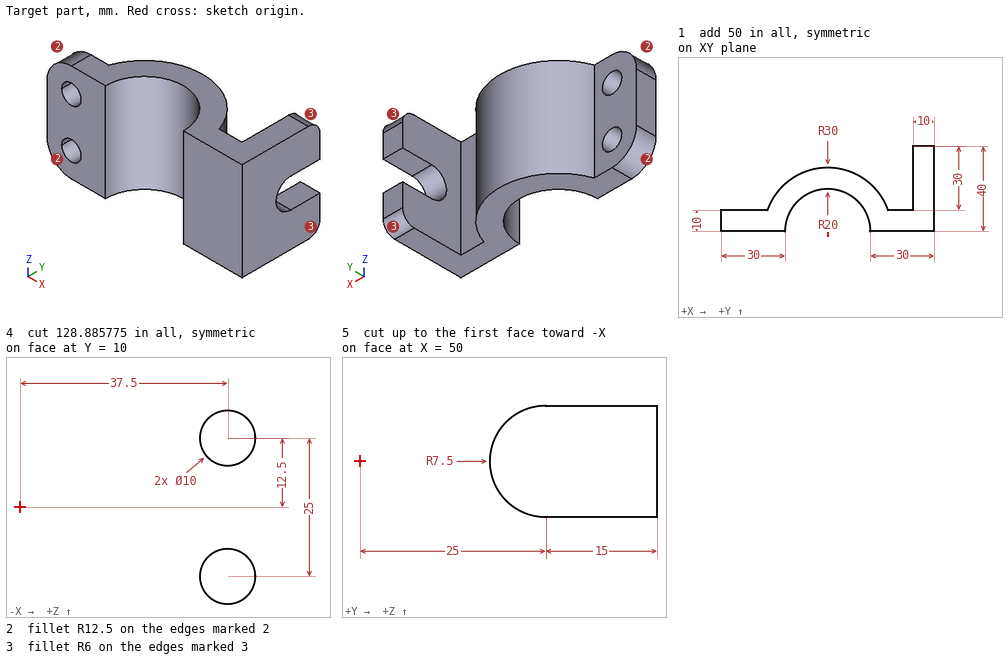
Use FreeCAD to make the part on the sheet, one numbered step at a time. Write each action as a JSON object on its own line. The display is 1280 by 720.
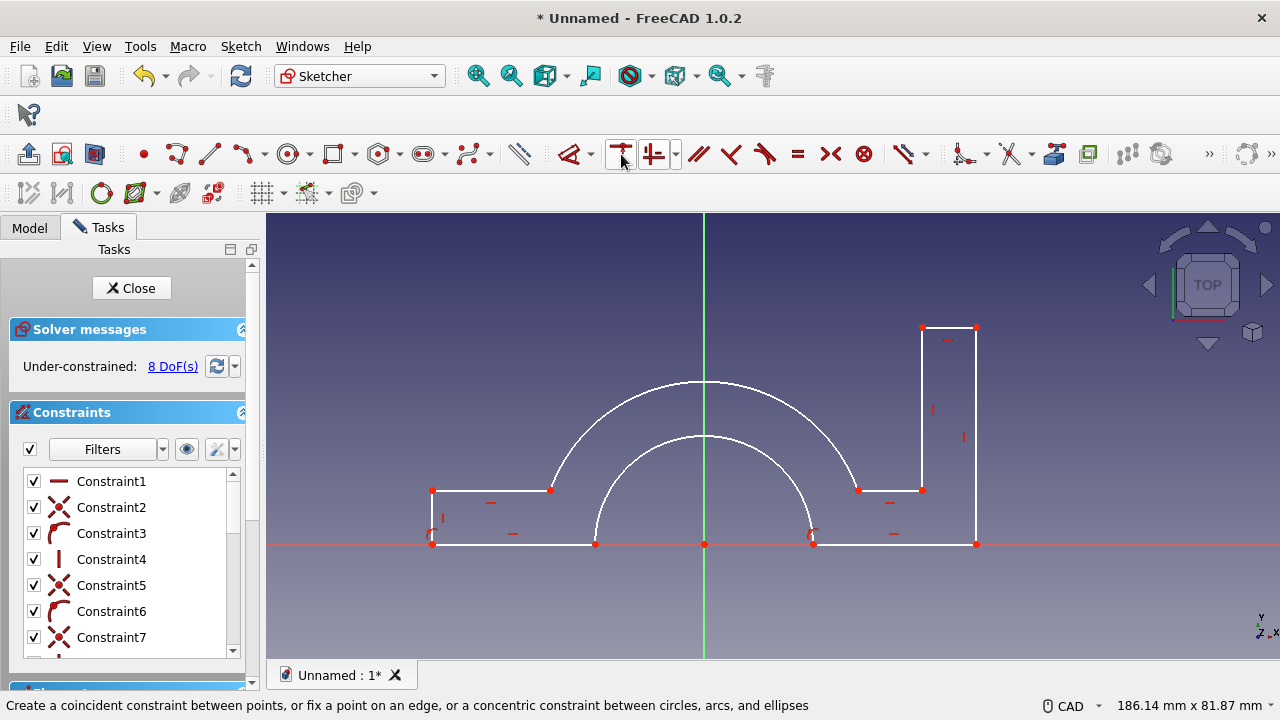
{"action": "left_click", "coordinate": [768, 457]}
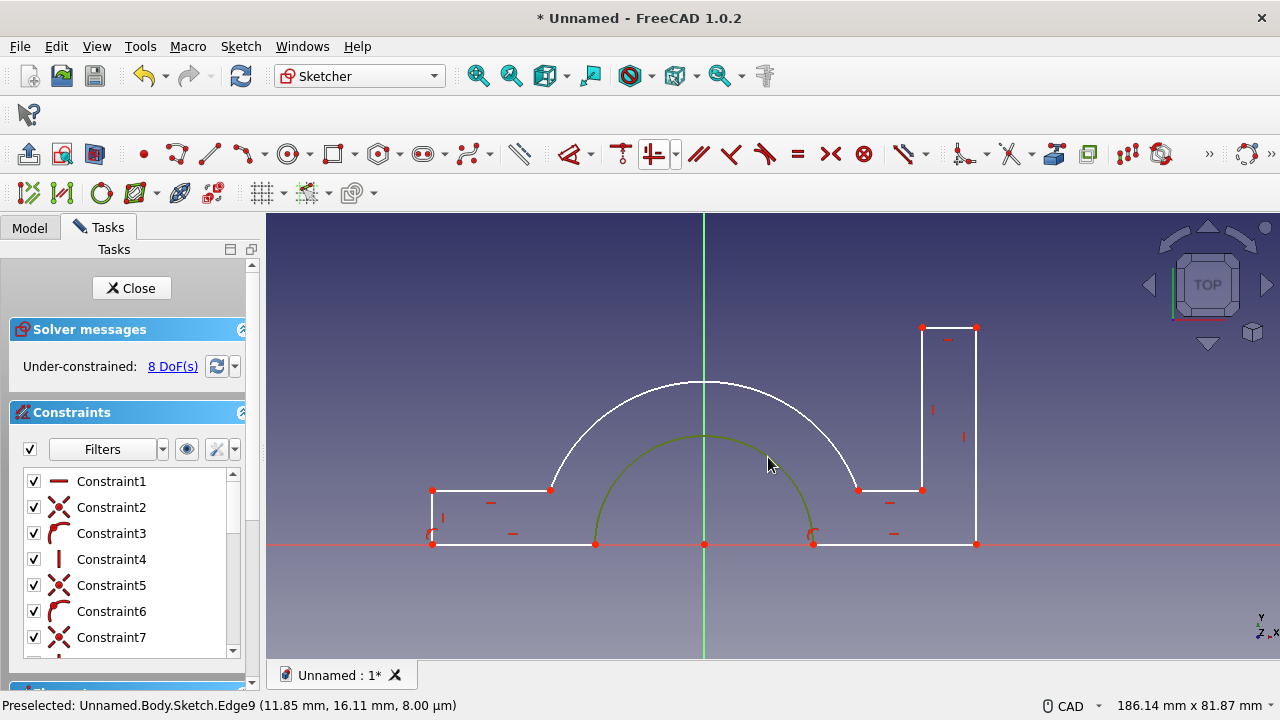
{"action": "key", "text": "k r"}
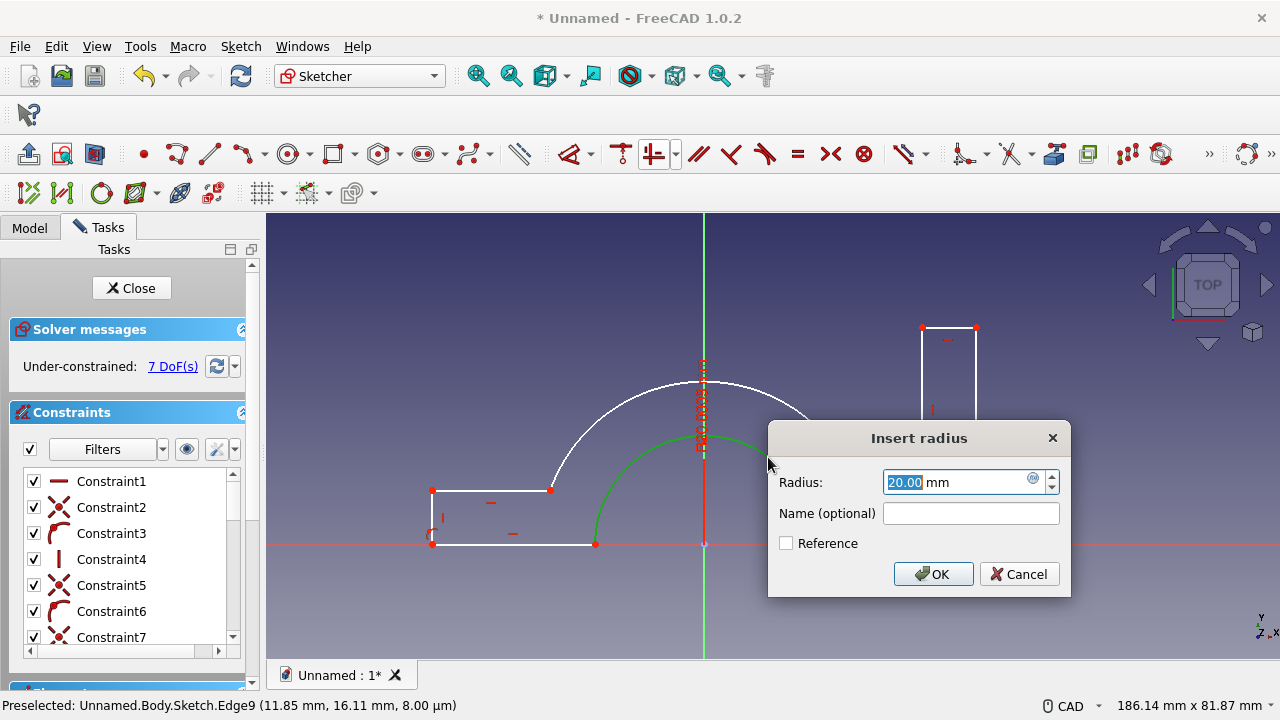
{"action": "type", "text": "20"}
{"action": "key", "text": "Return"}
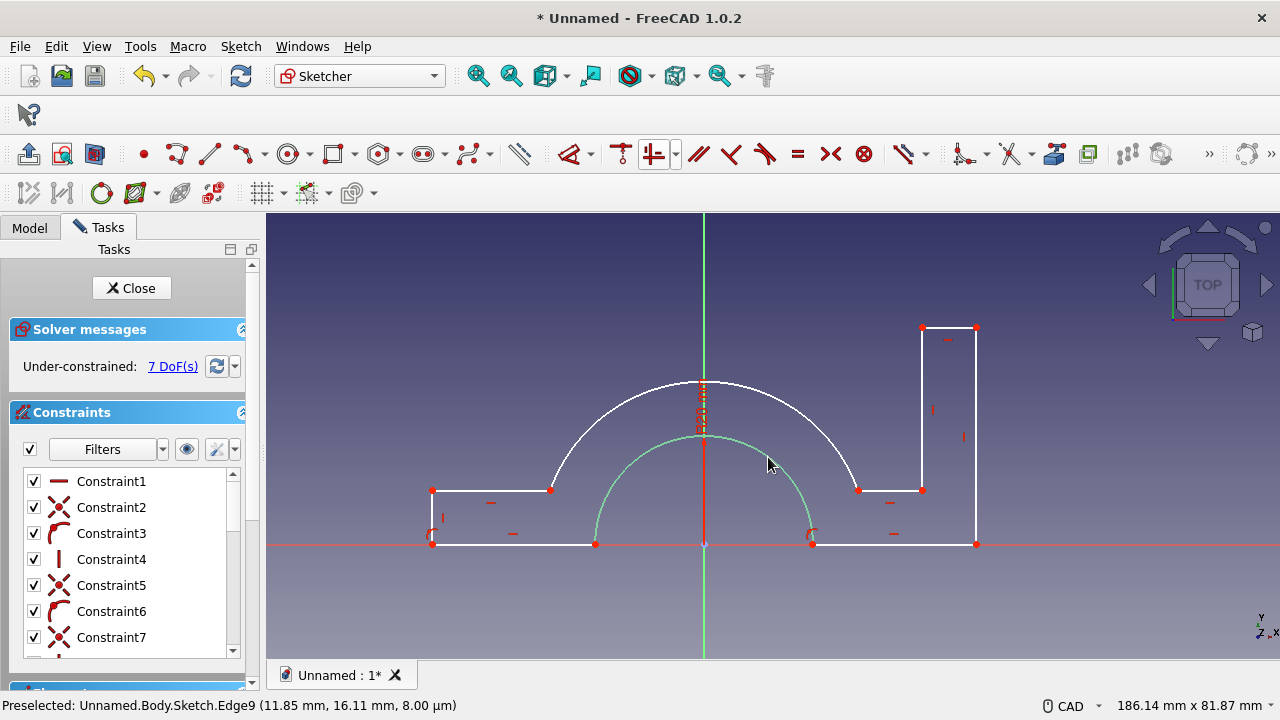
{"action": "left_click", "coordinate": [781, 401]}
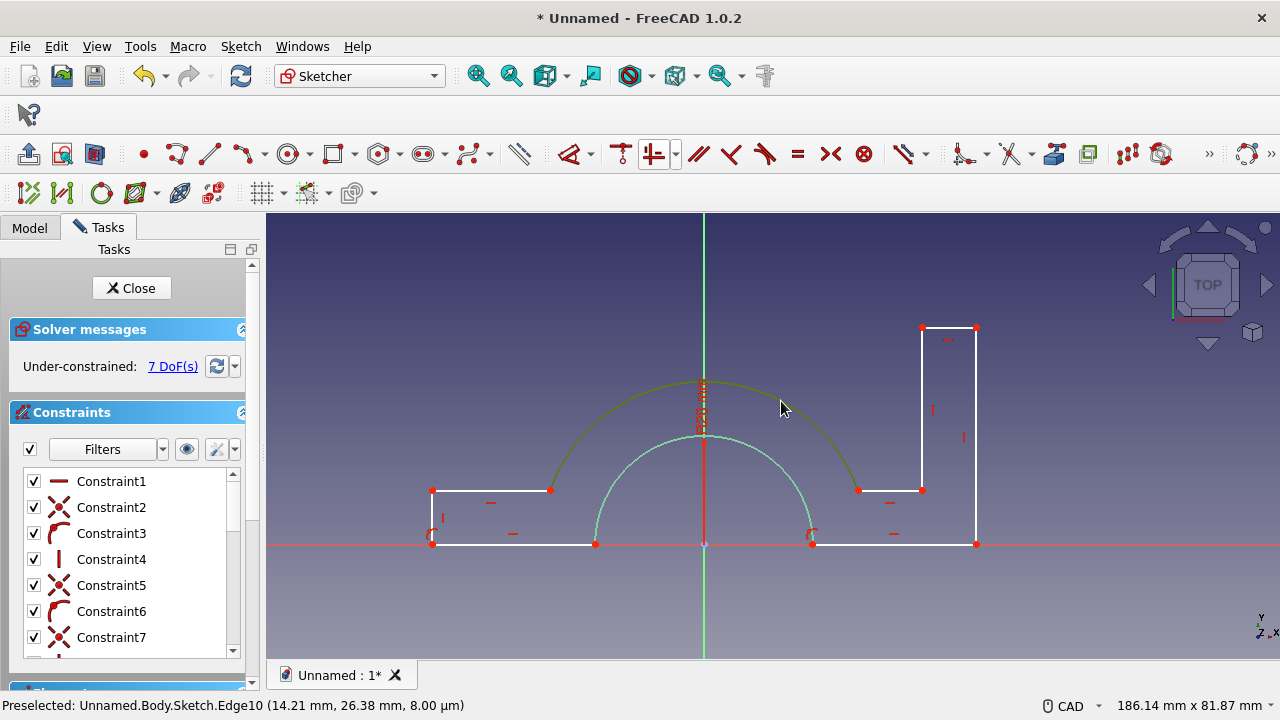
{"action": "left_click", "coordinate": [590, 154]}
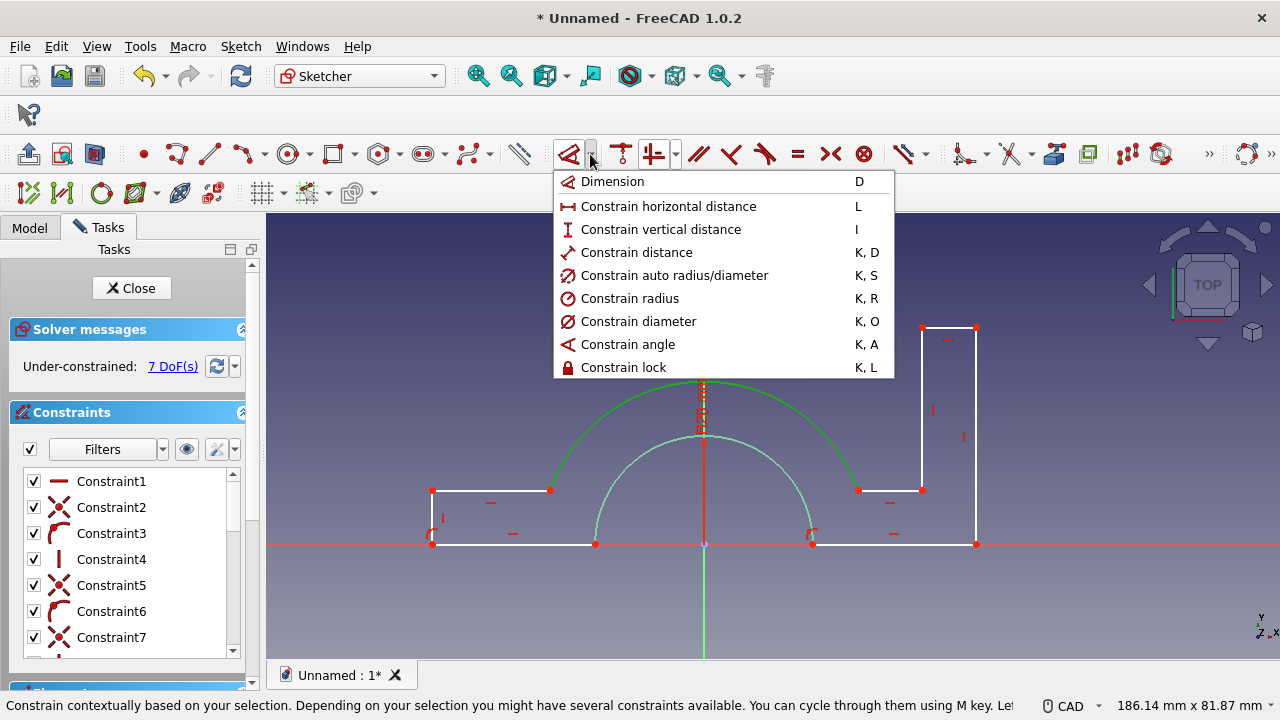
{"action": "left_click", "coordinate": [724, 298]}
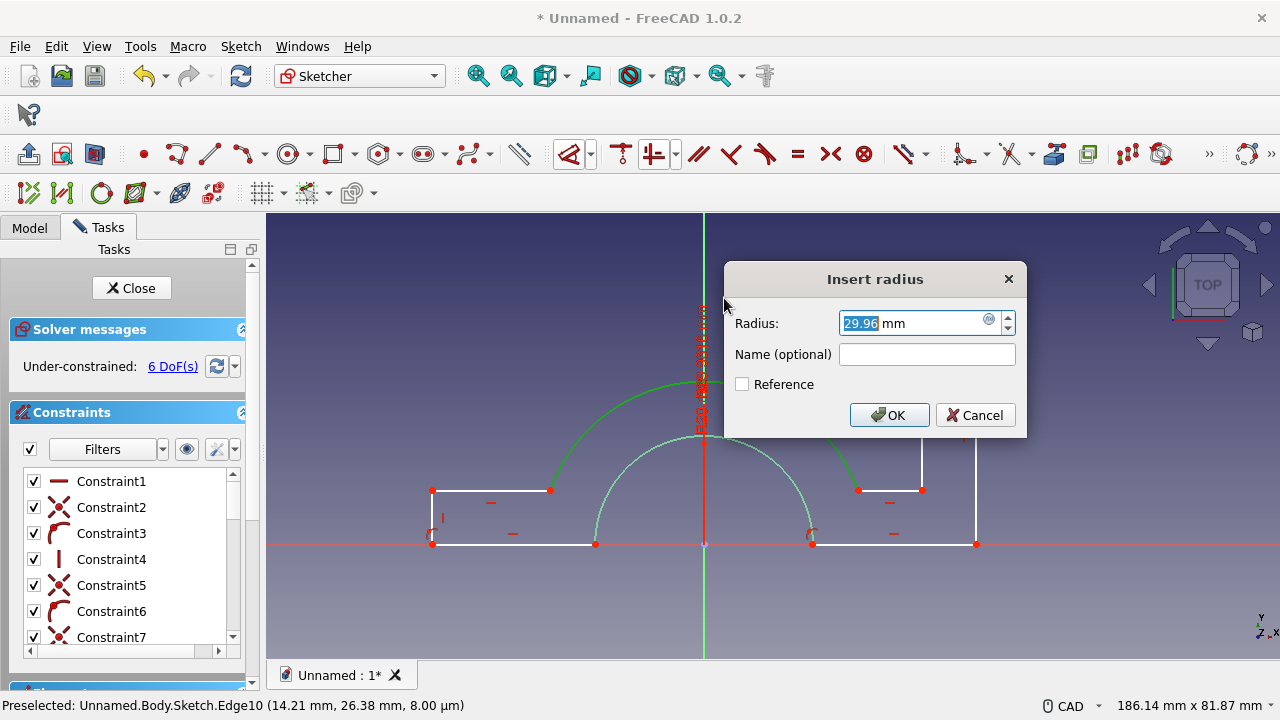
{"action": "type", "text": "30"}
{"action": "key", "text": "Return"}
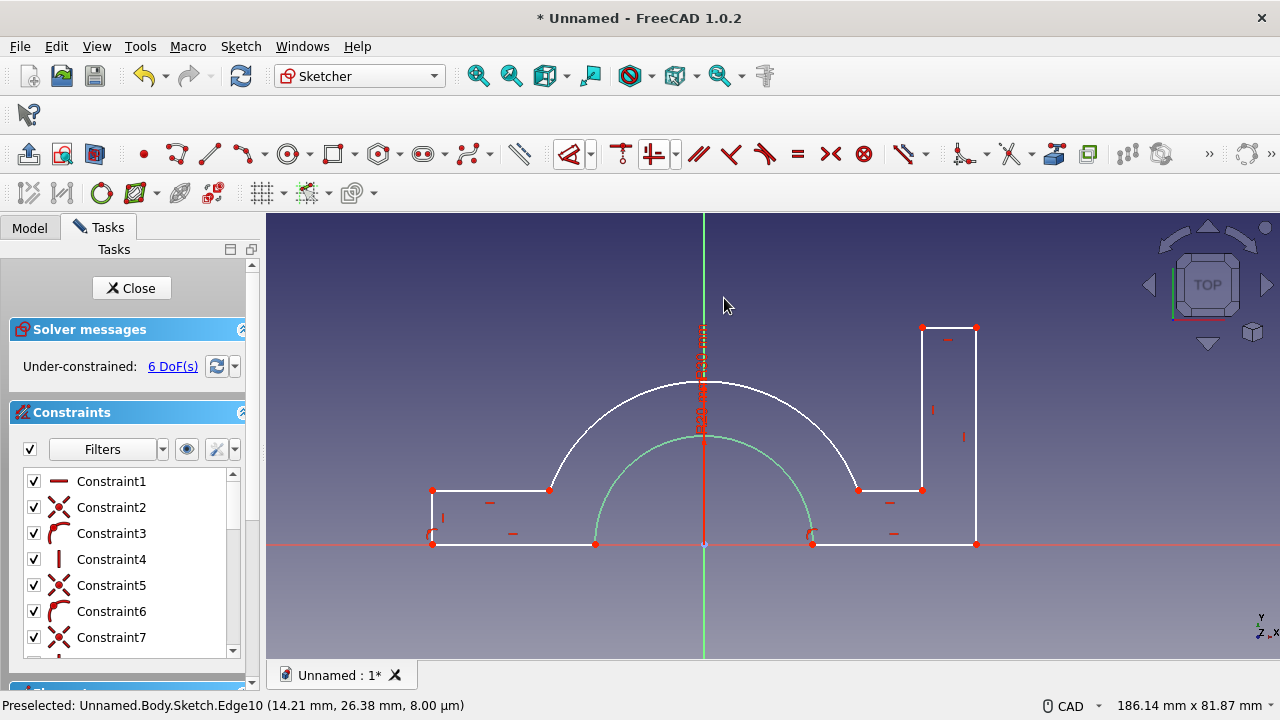
{"action": "left_click", "coordinate": [432, 507]}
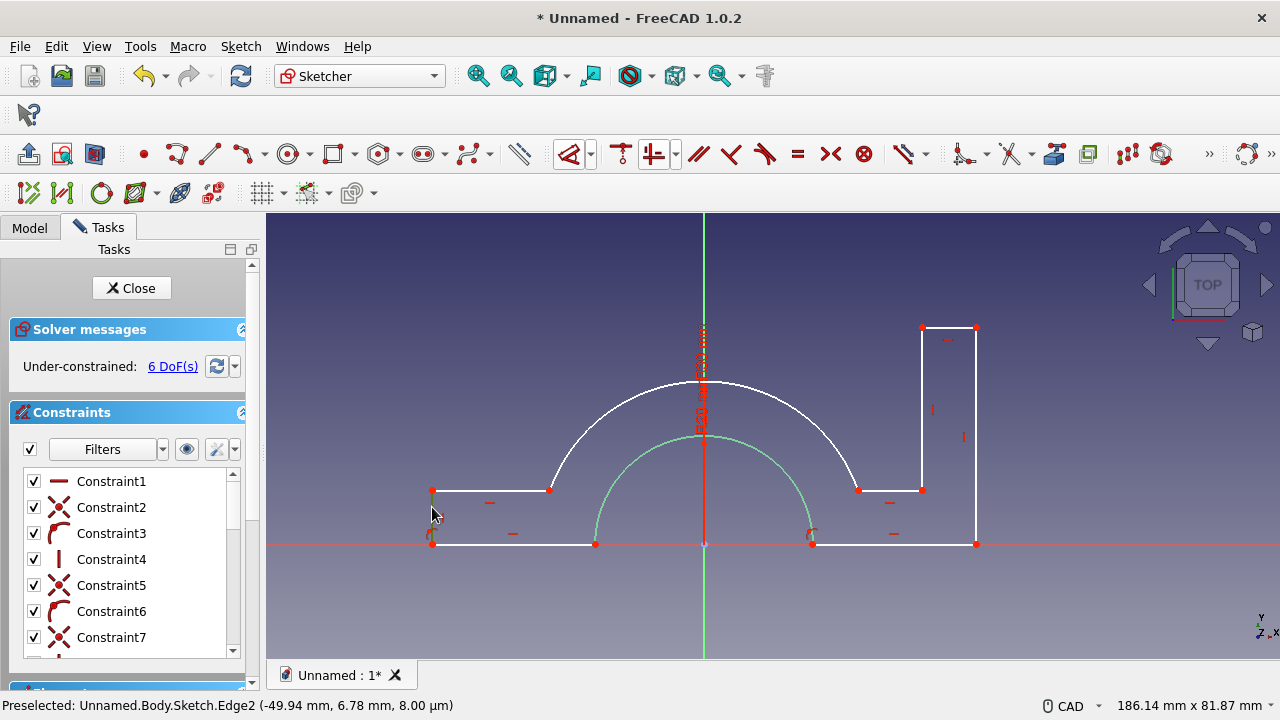
{"action": "key", "text": "i"}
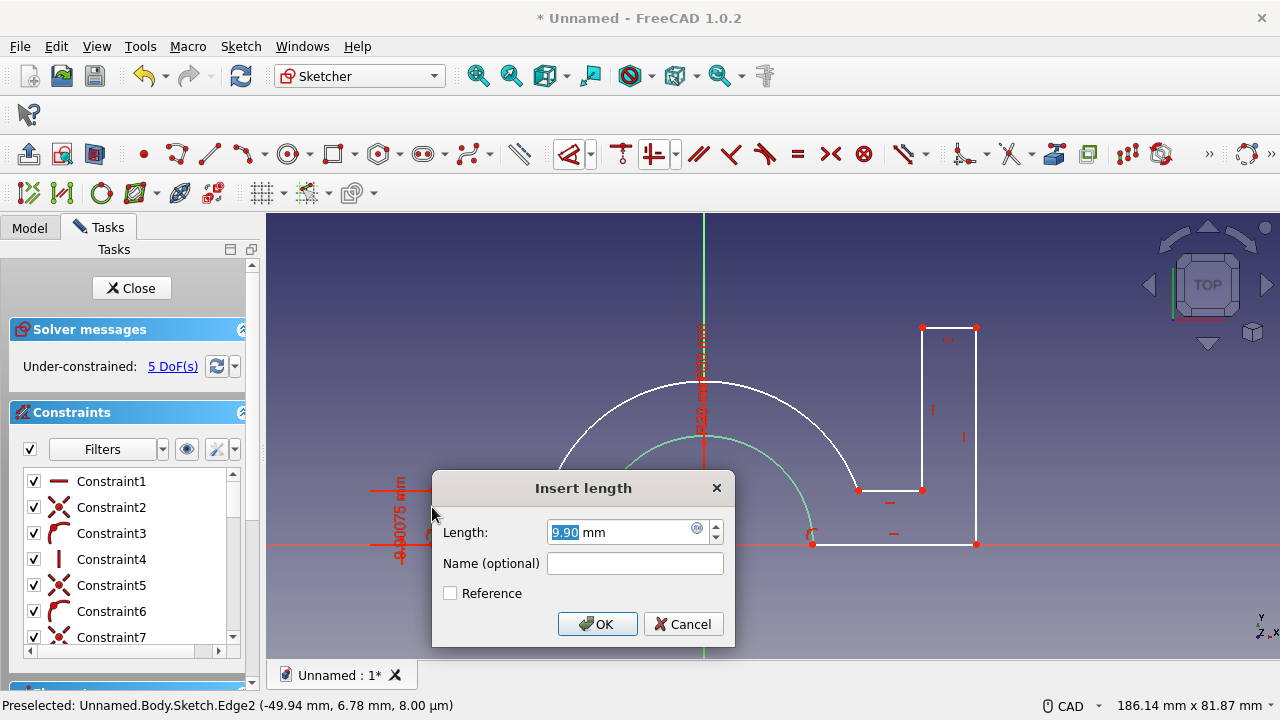
{"action": "type", "text": "10"}
{"action": "key", "text": "Return"}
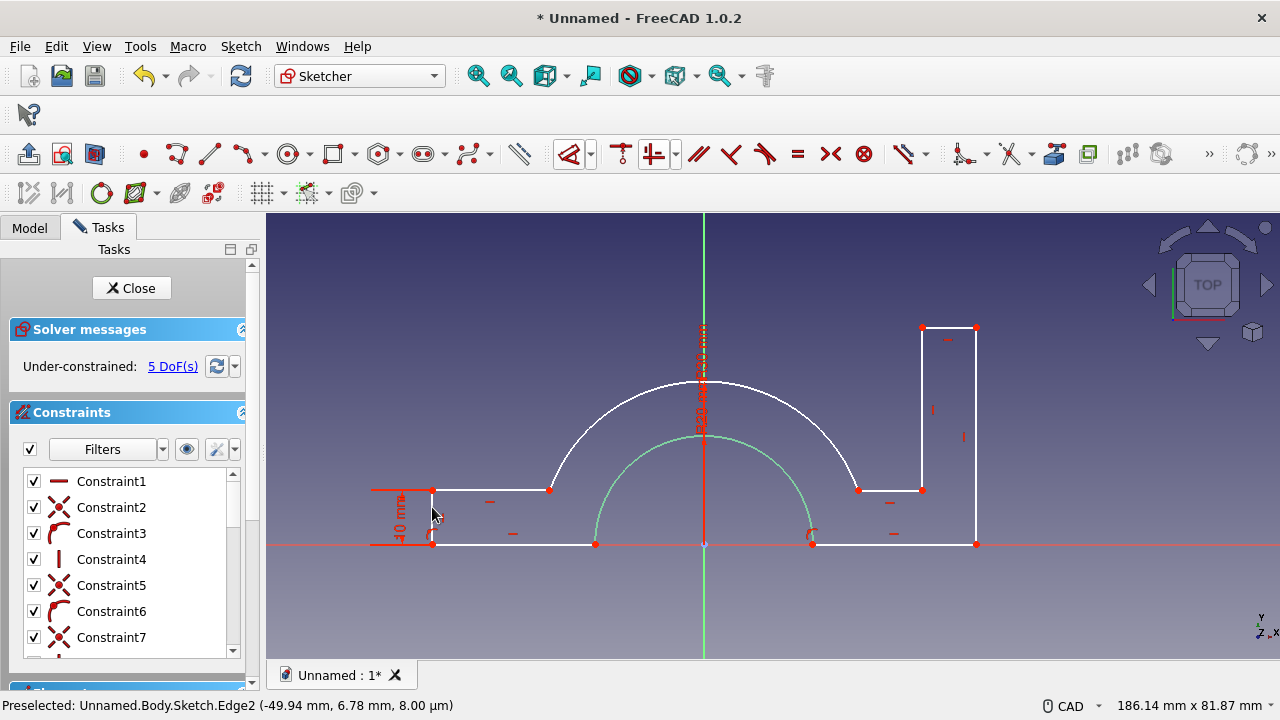
{"action": "left_click", "coordinate": [481, 545]}